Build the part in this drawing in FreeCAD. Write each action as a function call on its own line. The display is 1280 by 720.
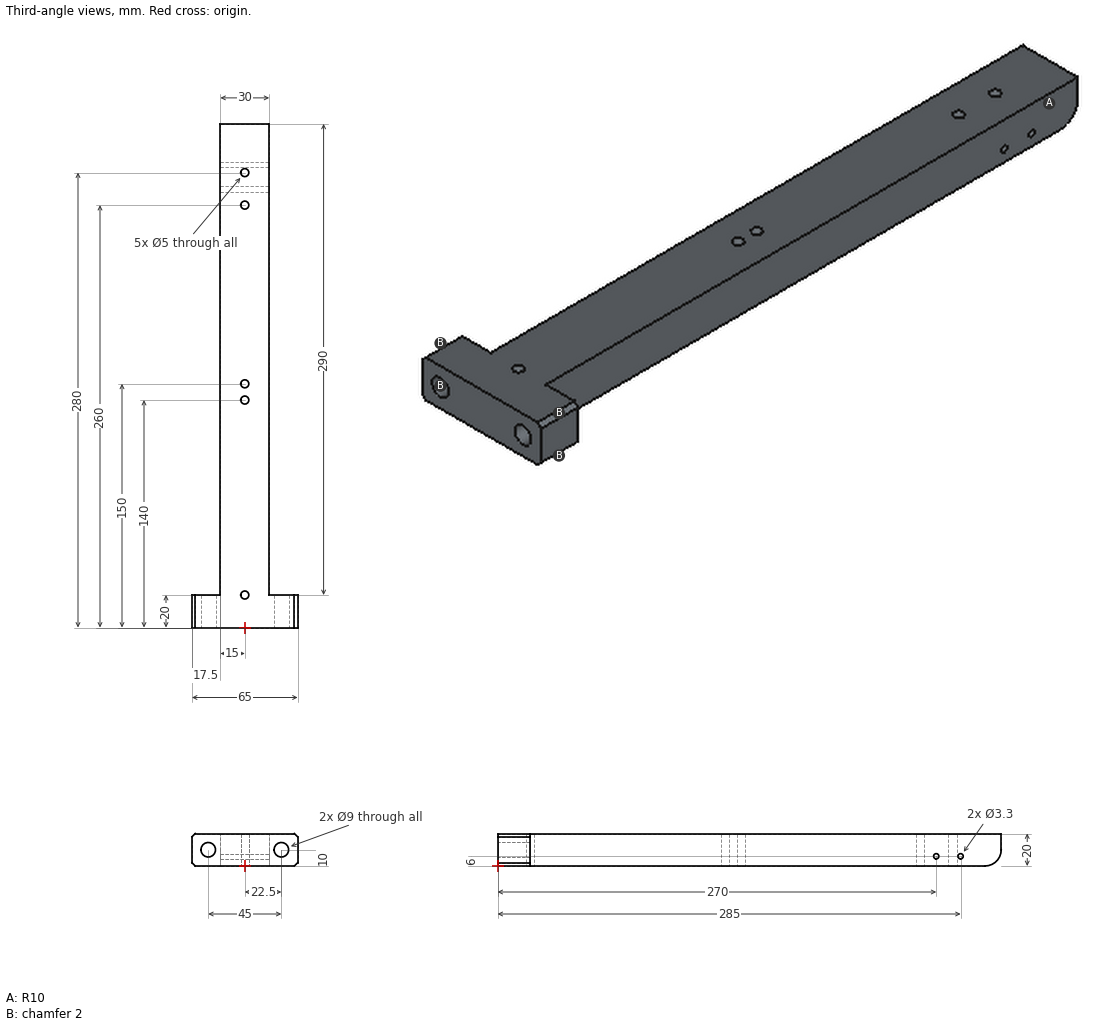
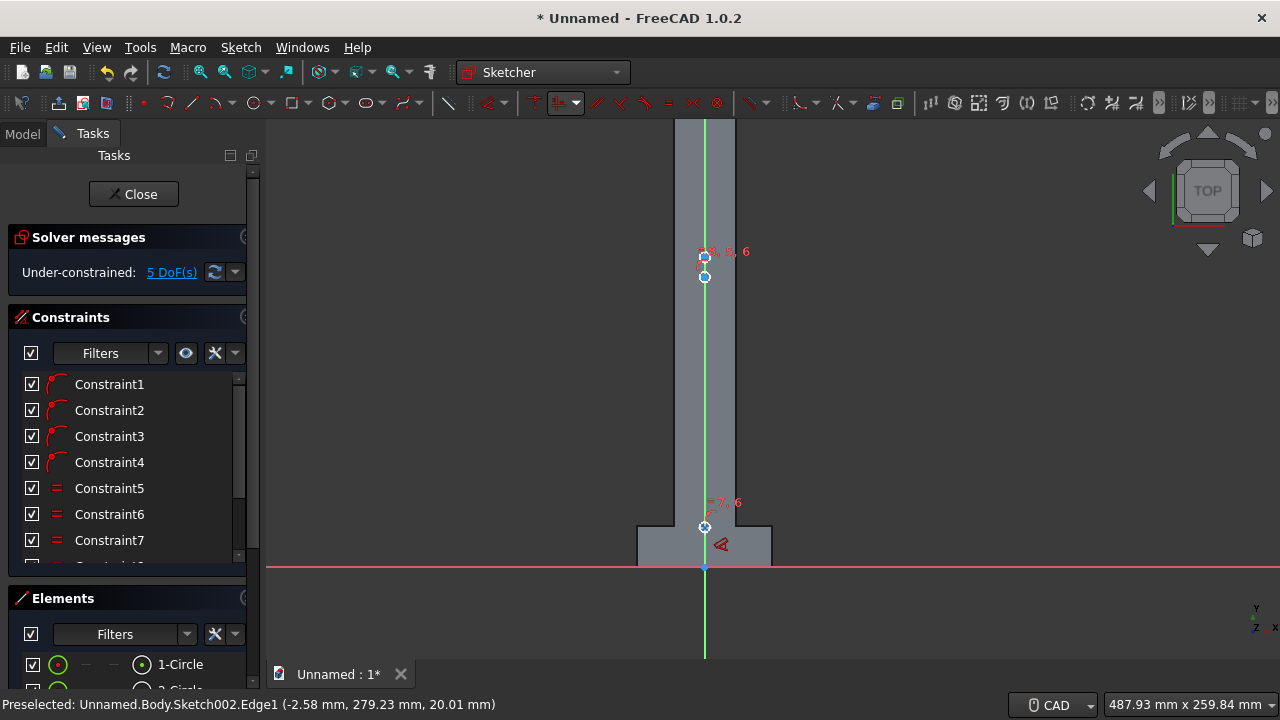
click(705, 527)
click(739, 547)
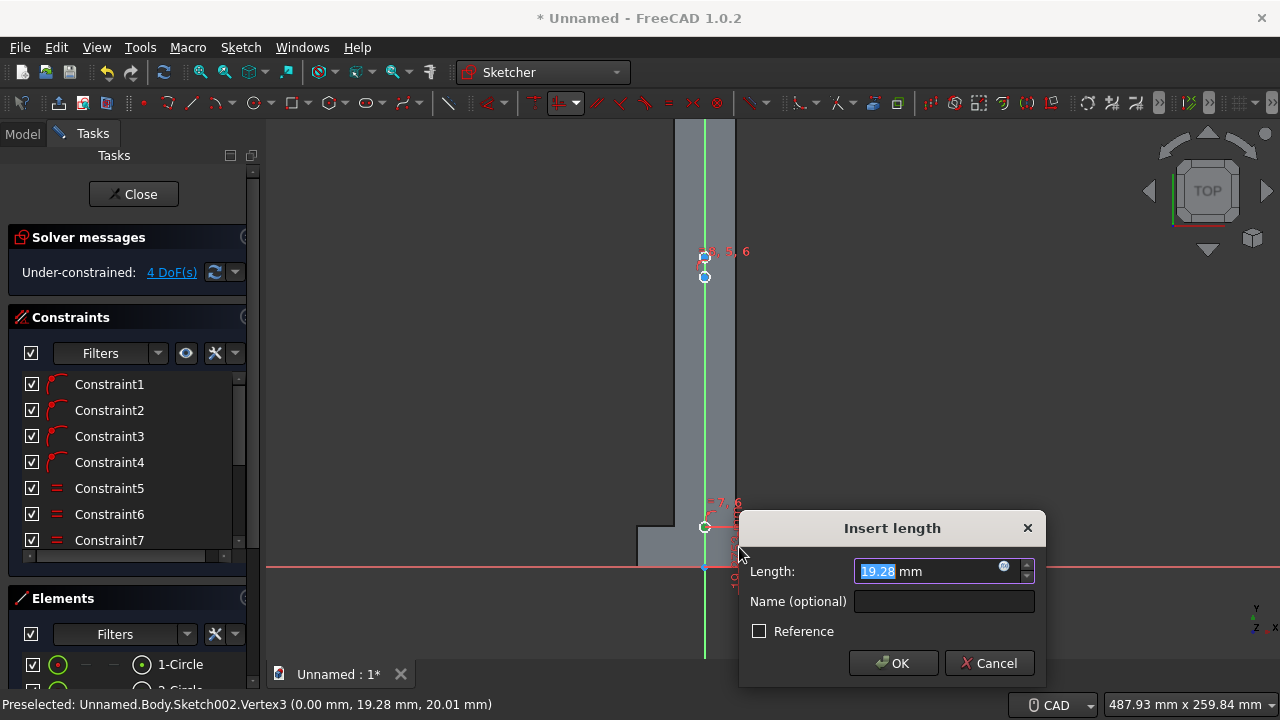
text(20)
key(Return)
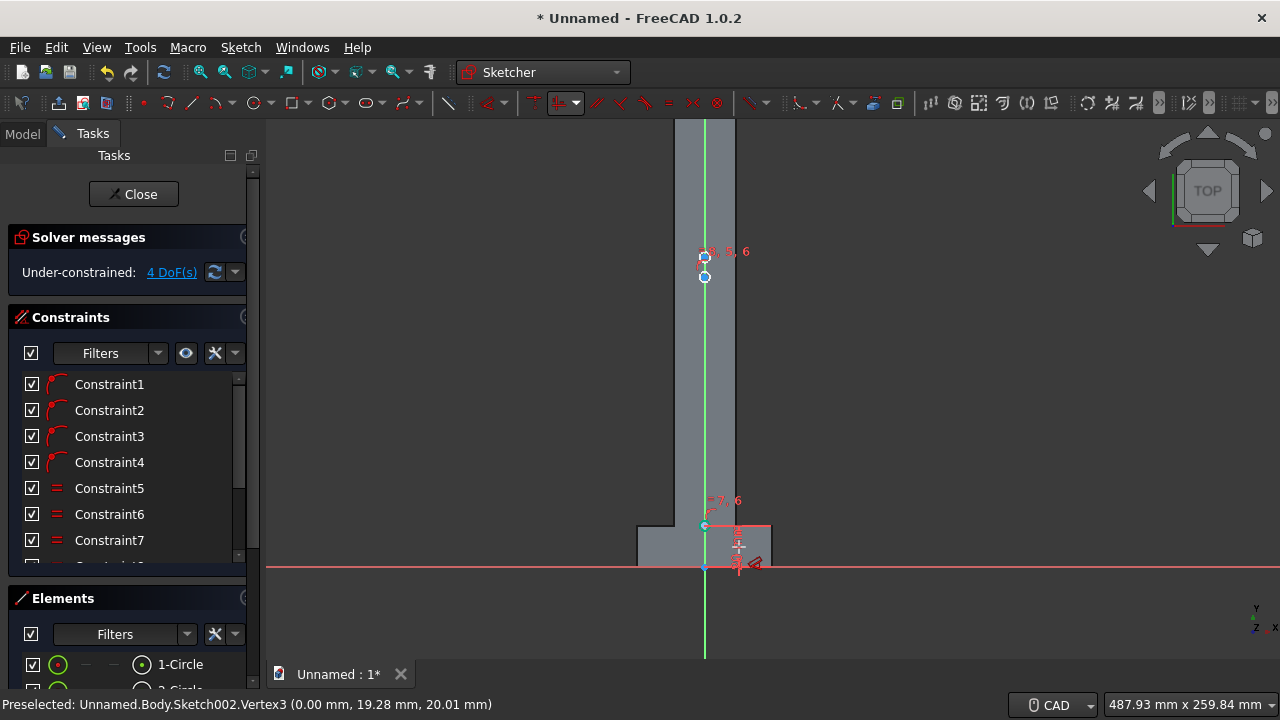
scroll(704, 529, down, 3)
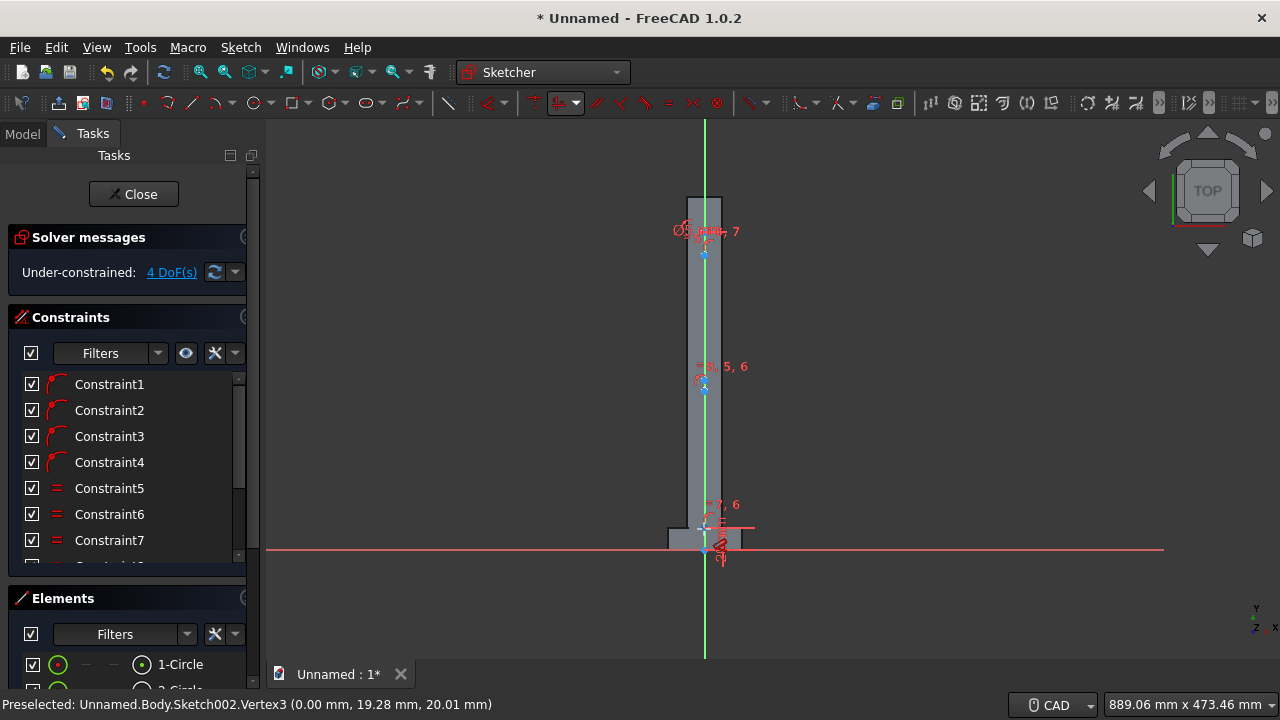
click(705, 232)
click(739, 391)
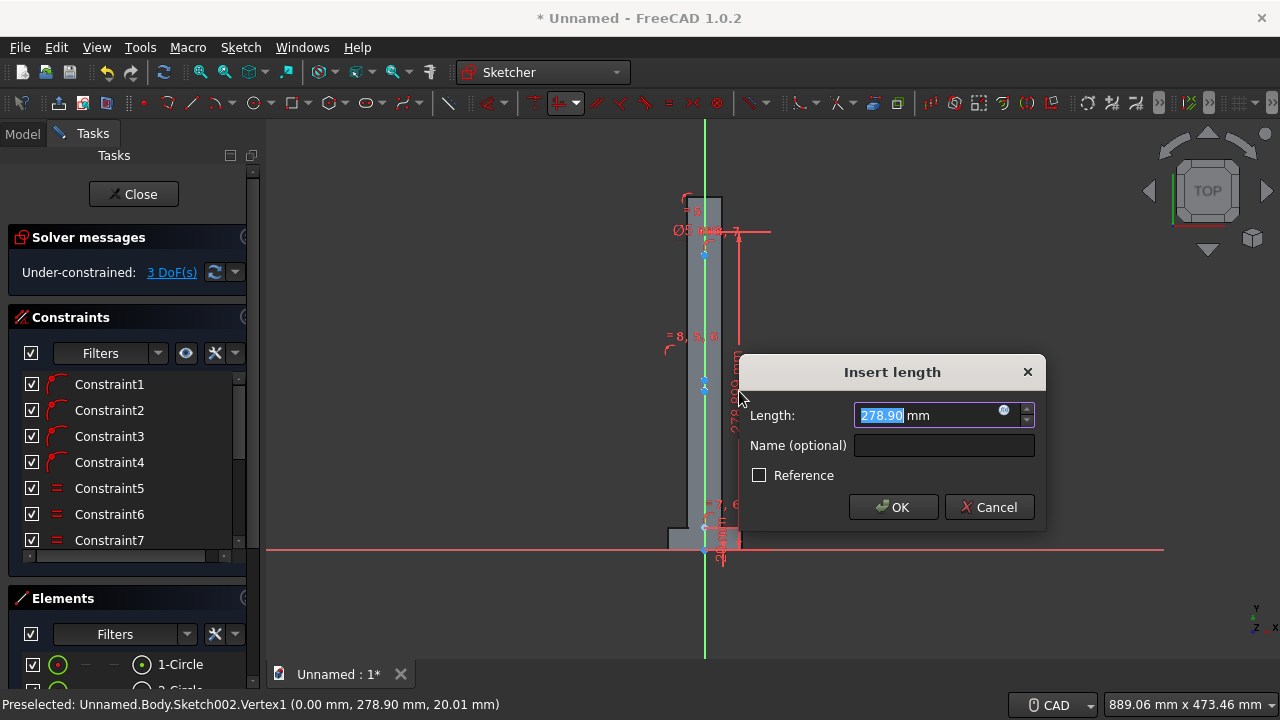
text(280)
key(Return)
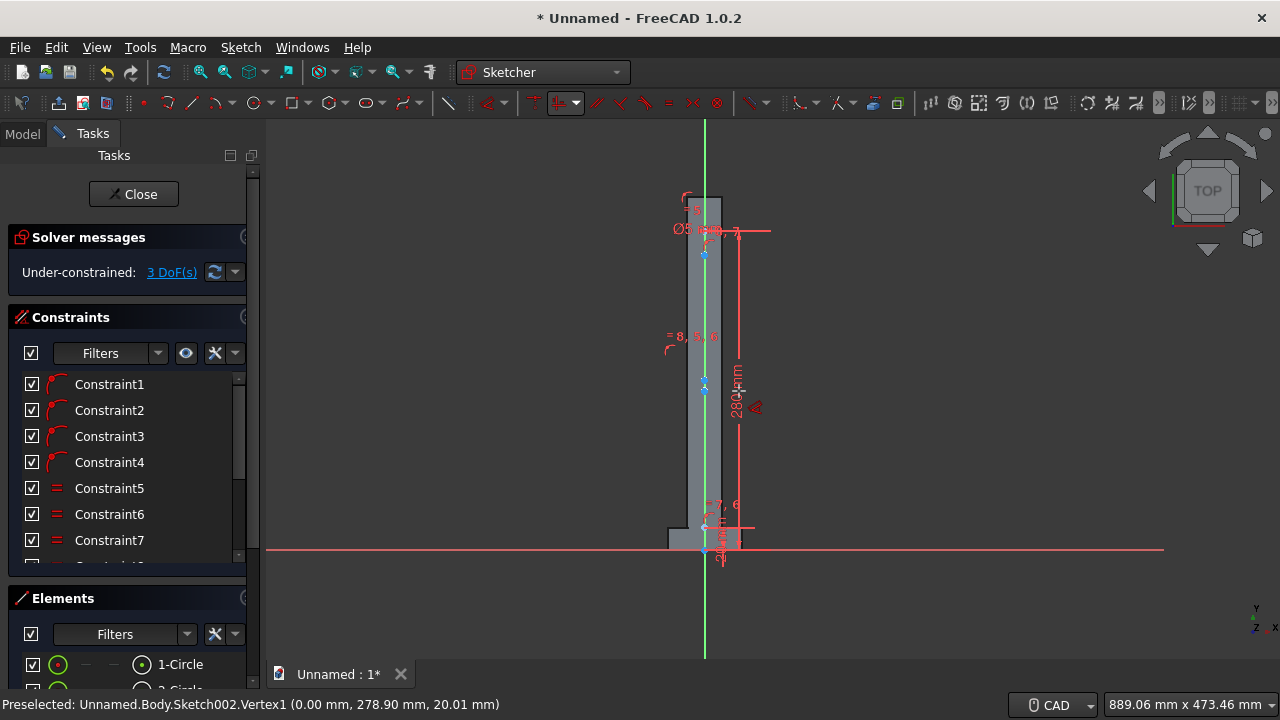
click(705, 380)
click(739, 465)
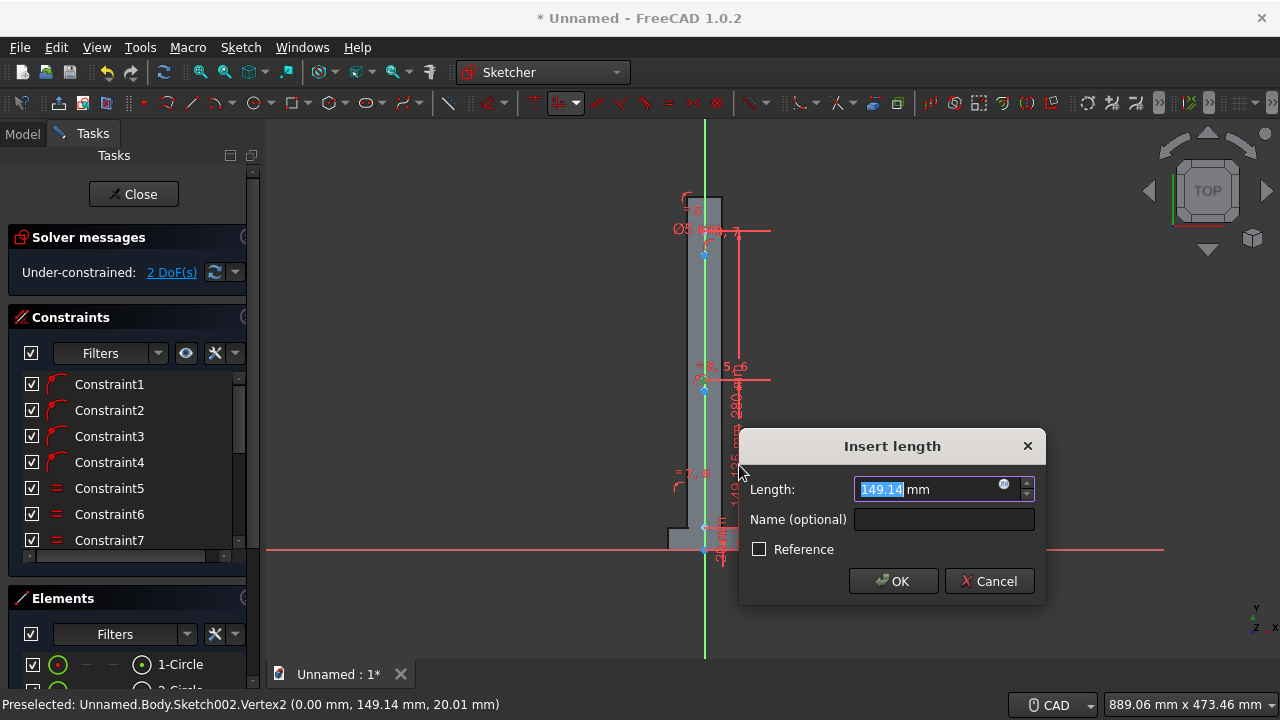
text(150)
key(Return)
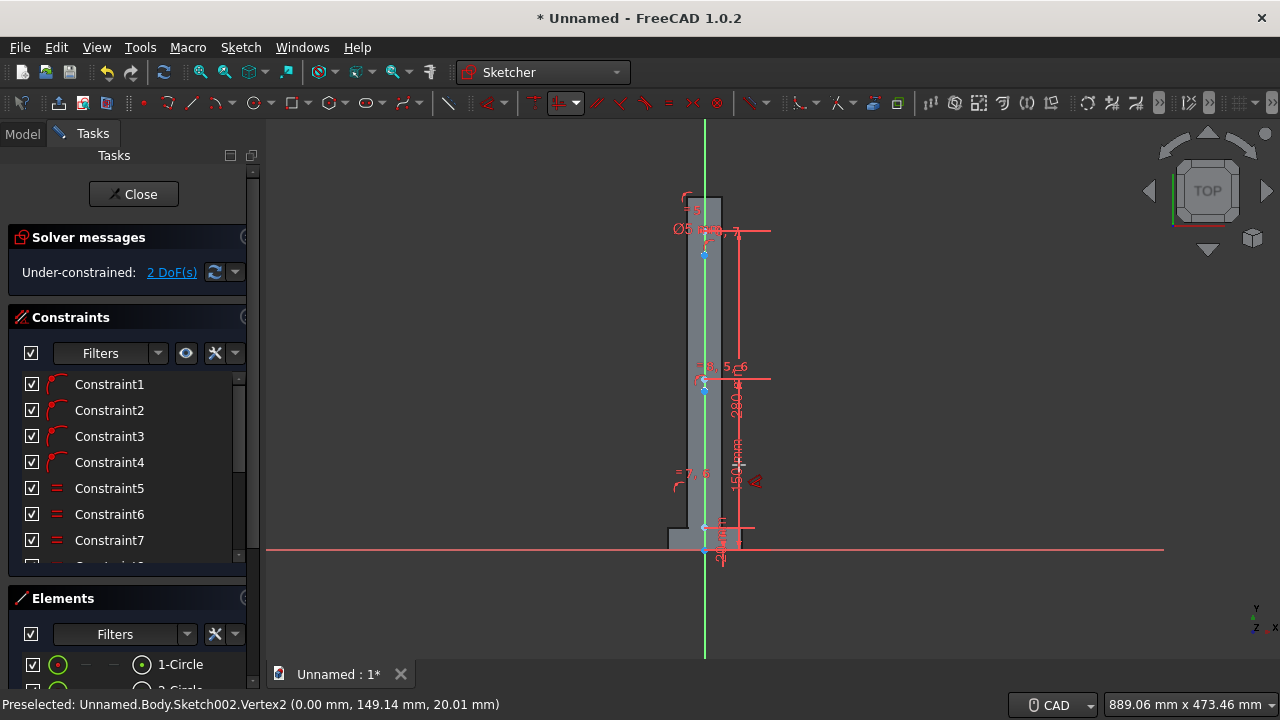
click(705, 255)
click(739, 335)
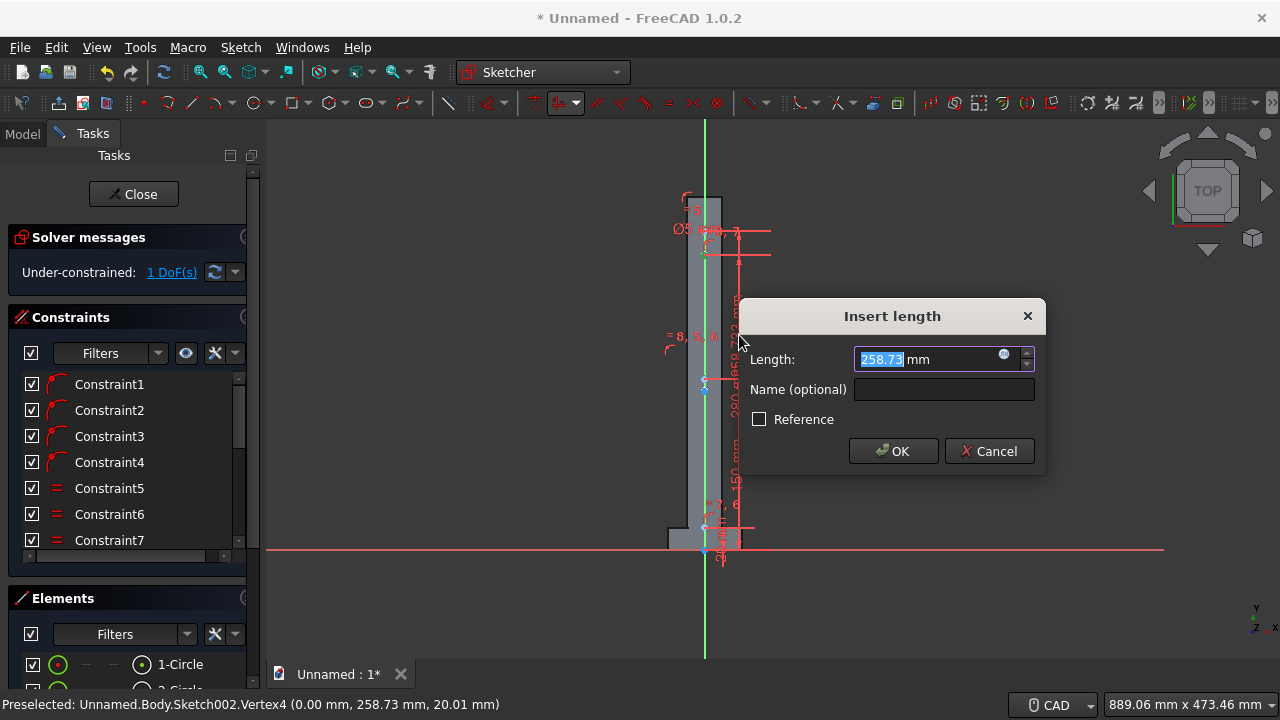
text(260)
key(Return)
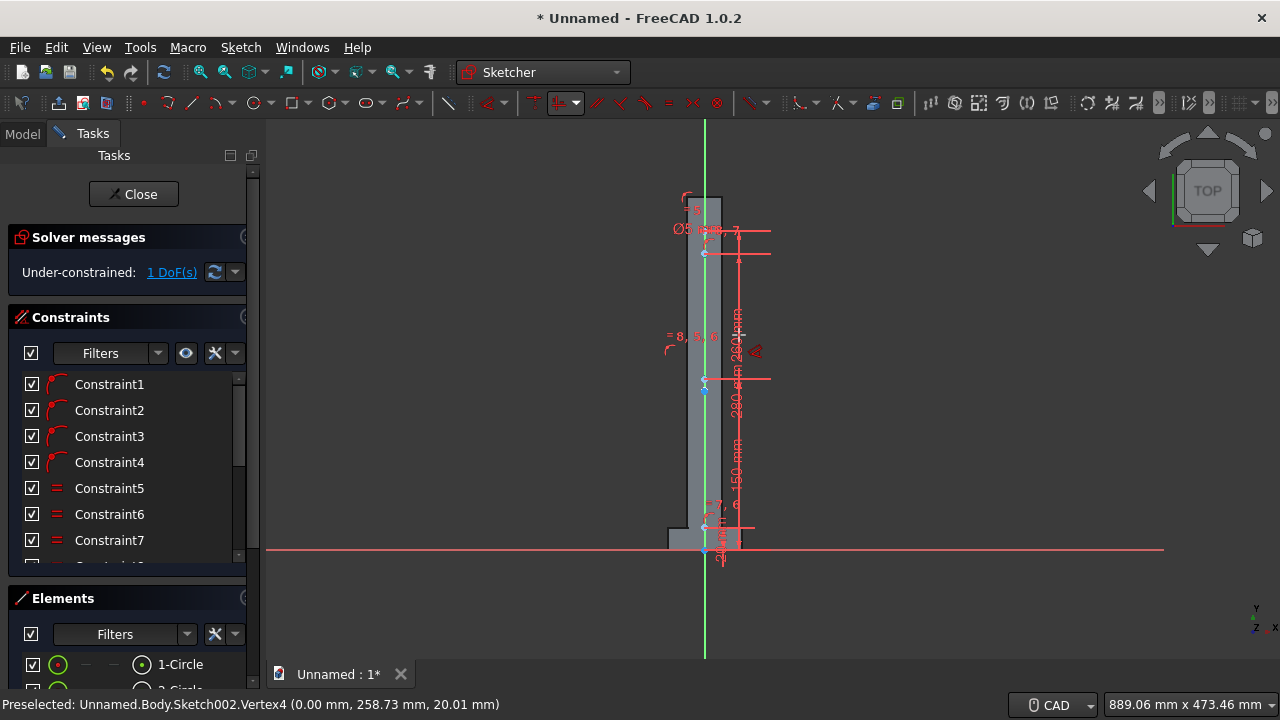
click(705, 391)
click(739, 434)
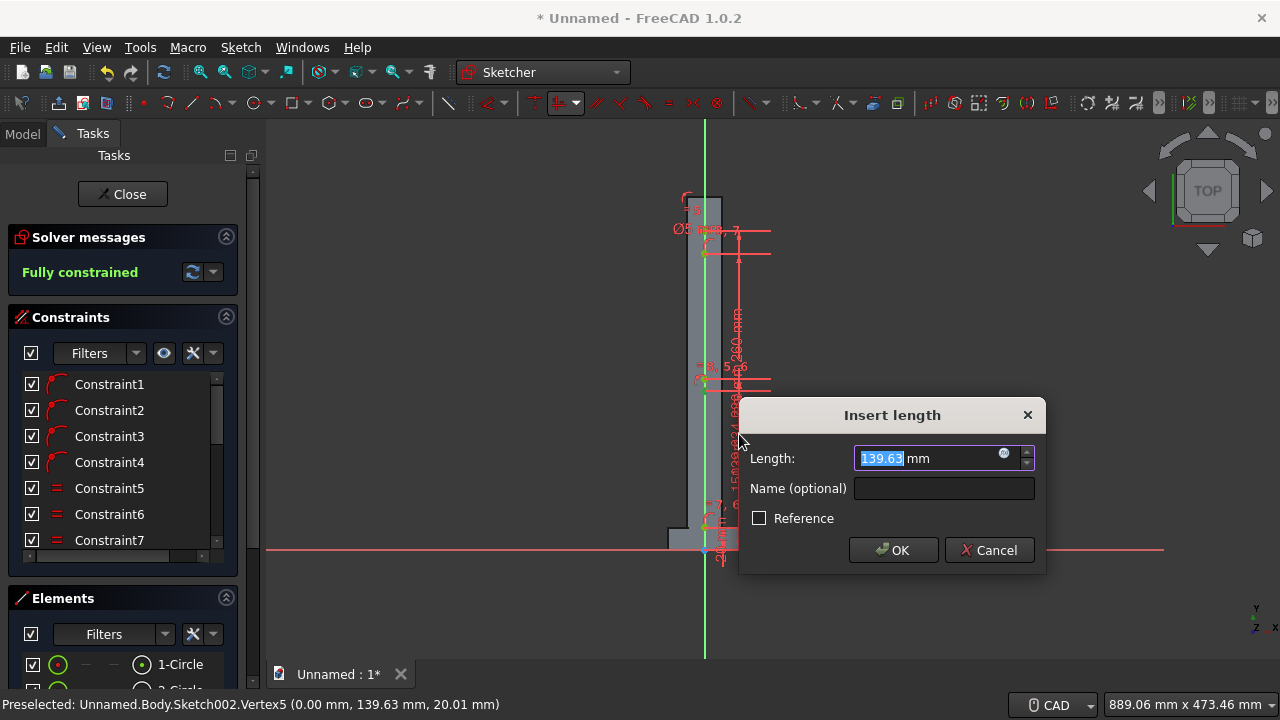
text(140)
key(Return)
key(Escape)